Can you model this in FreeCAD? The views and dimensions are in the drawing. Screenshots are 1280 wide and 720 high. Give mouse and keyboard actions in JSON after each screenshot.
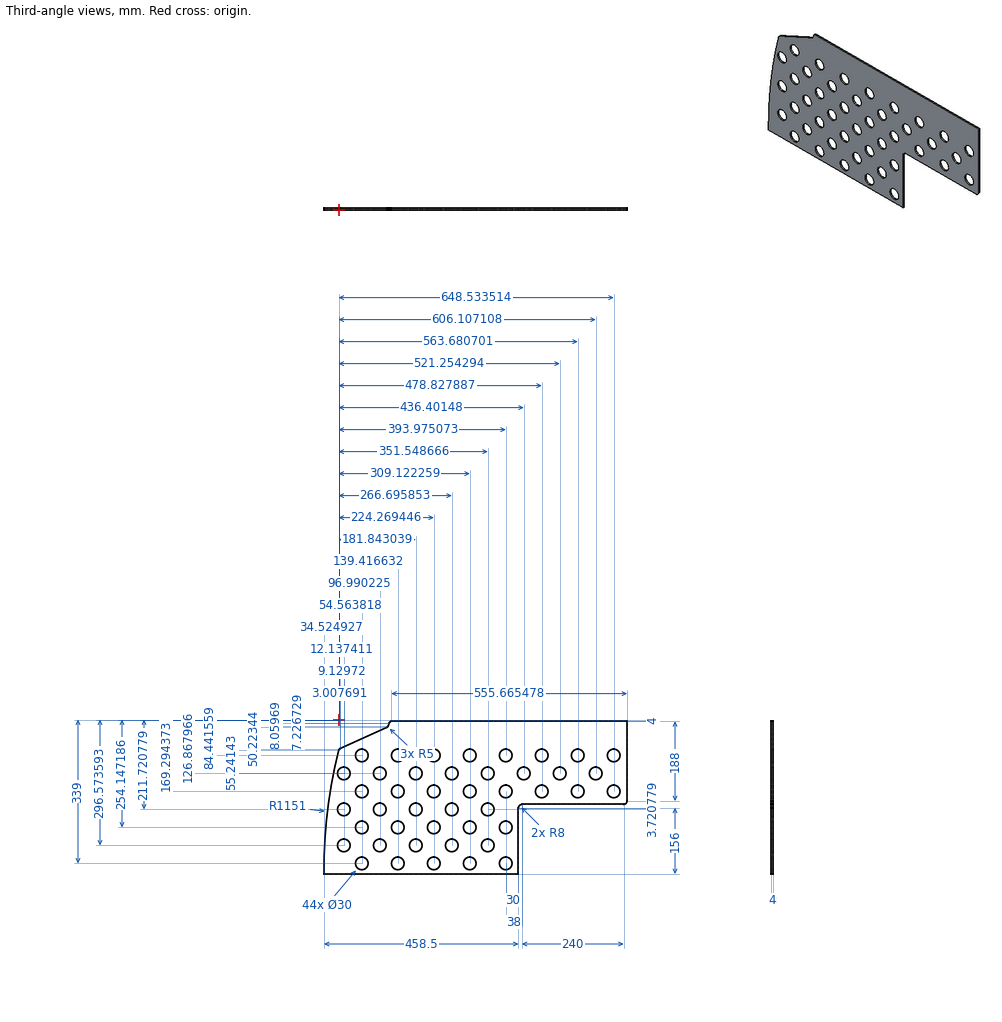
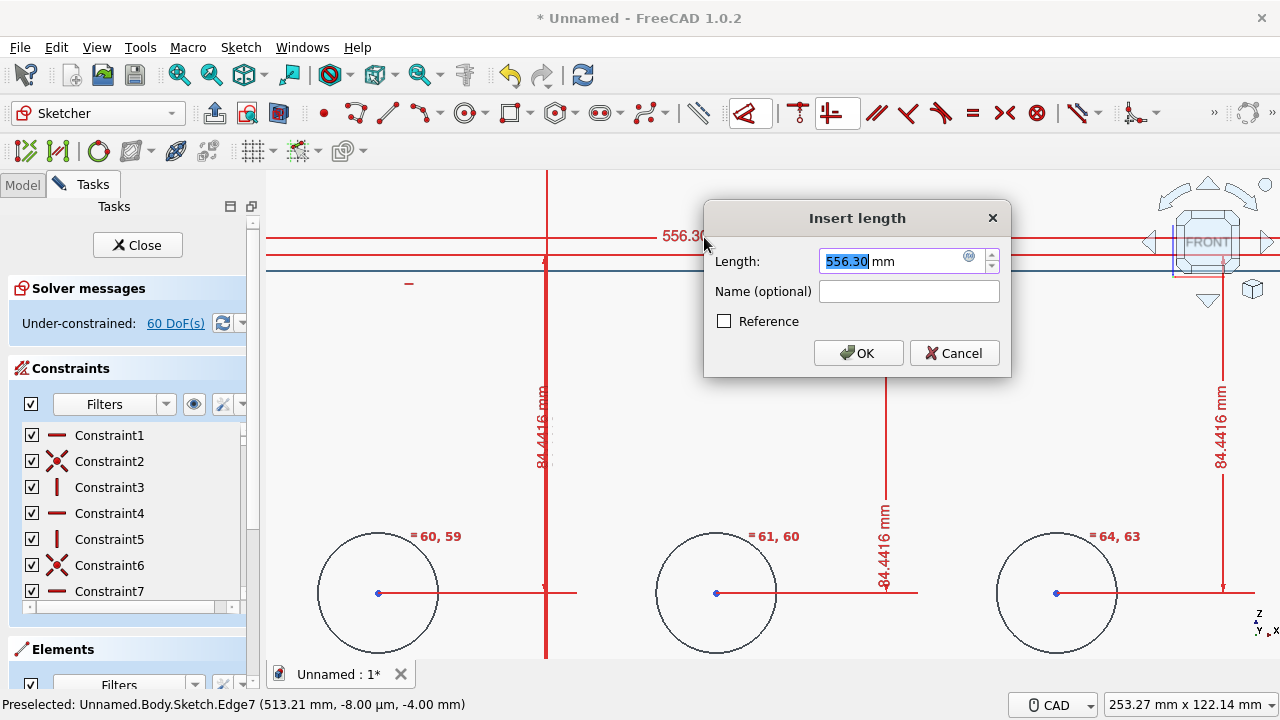
{"action": "type", "text": "555.665478"}
{"action": "key", "text": "Return"}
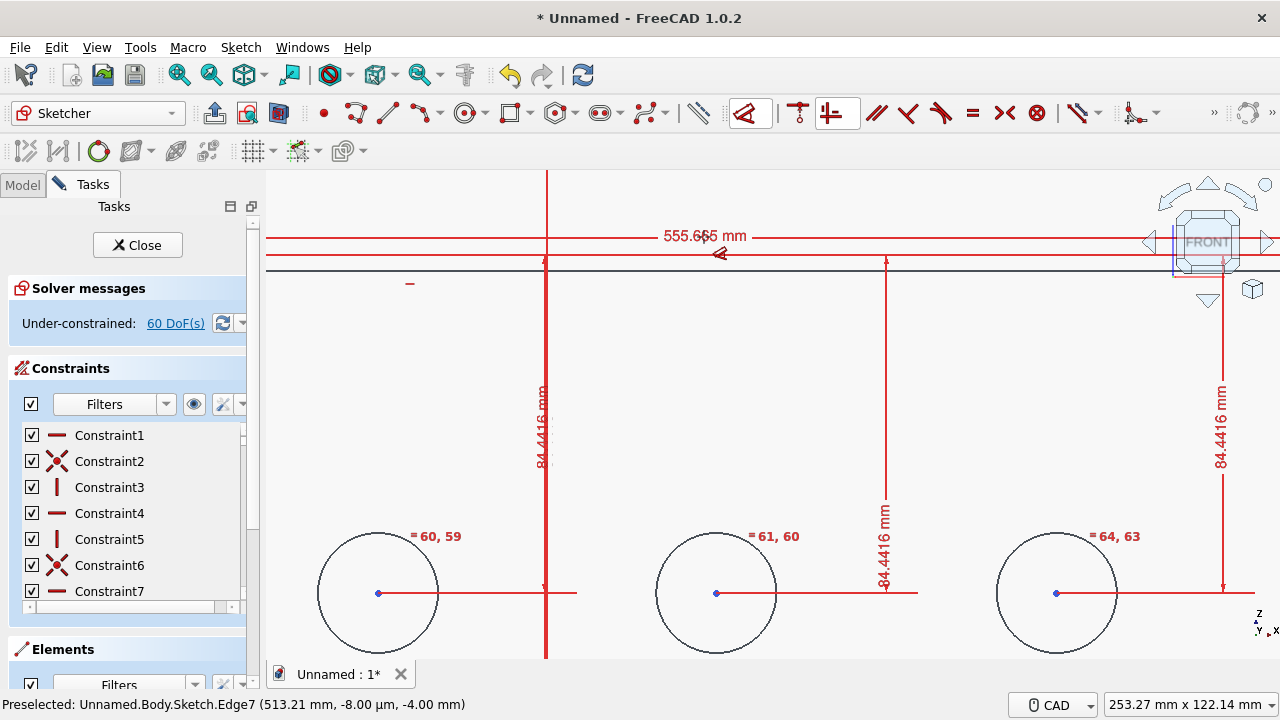
{"action": "scroll", "coordinate": [859, 271], "scroll_direction": "down", "scroll_amount": 8}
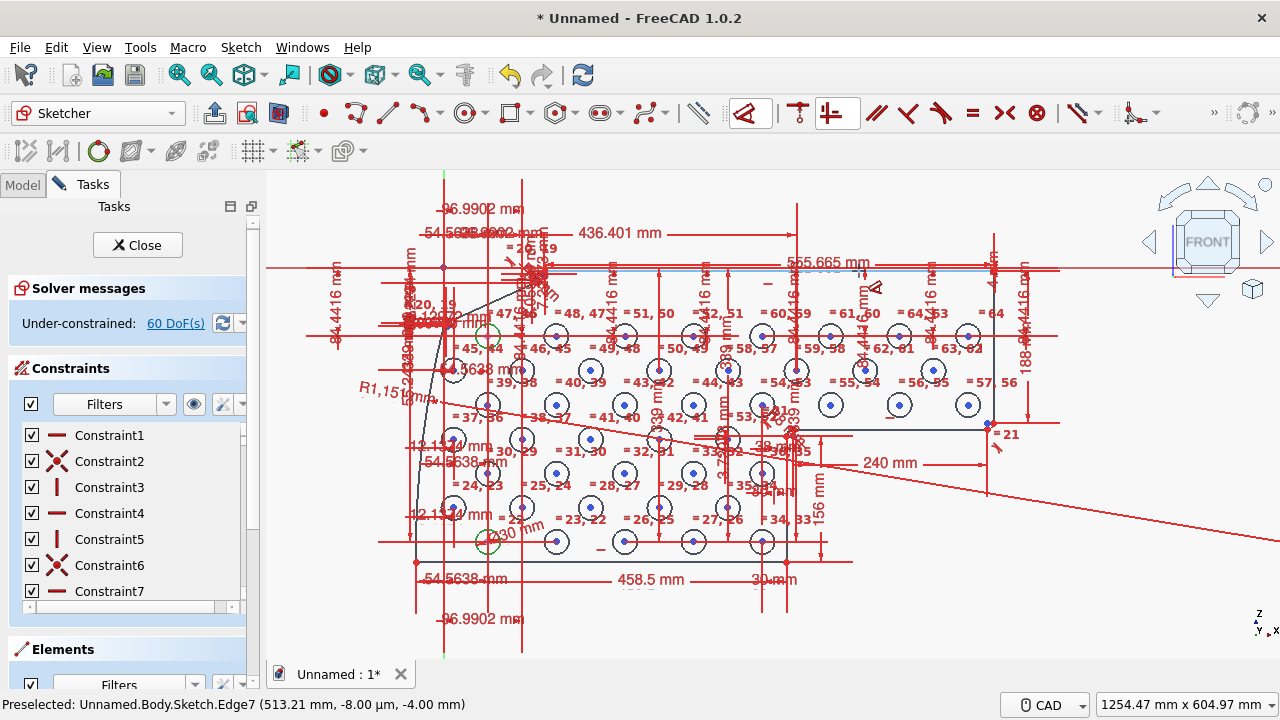
{"action": "scroll", "coordinate": [416, 562], "scroll_direction": "up", "scroll_amount": 2}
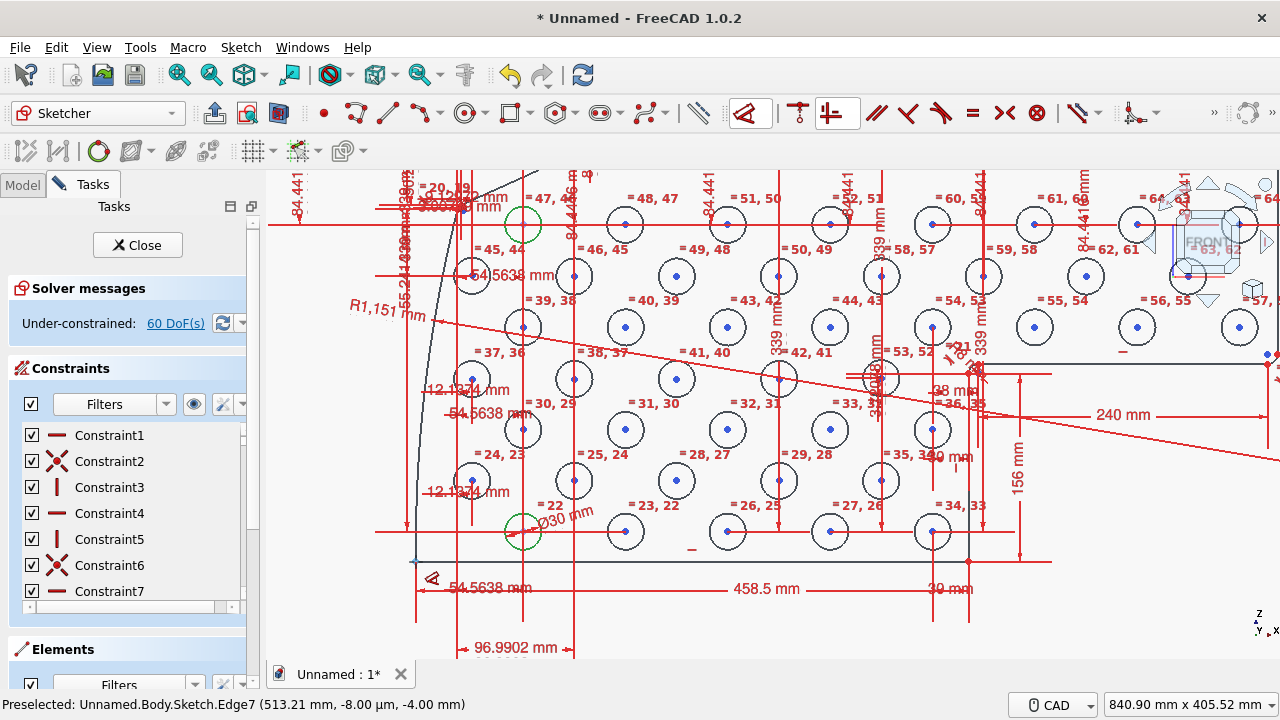
{"action": "left_click", "coordinate": [416, 562]}
{"action": "left_click", "coordinate": [437, 620]}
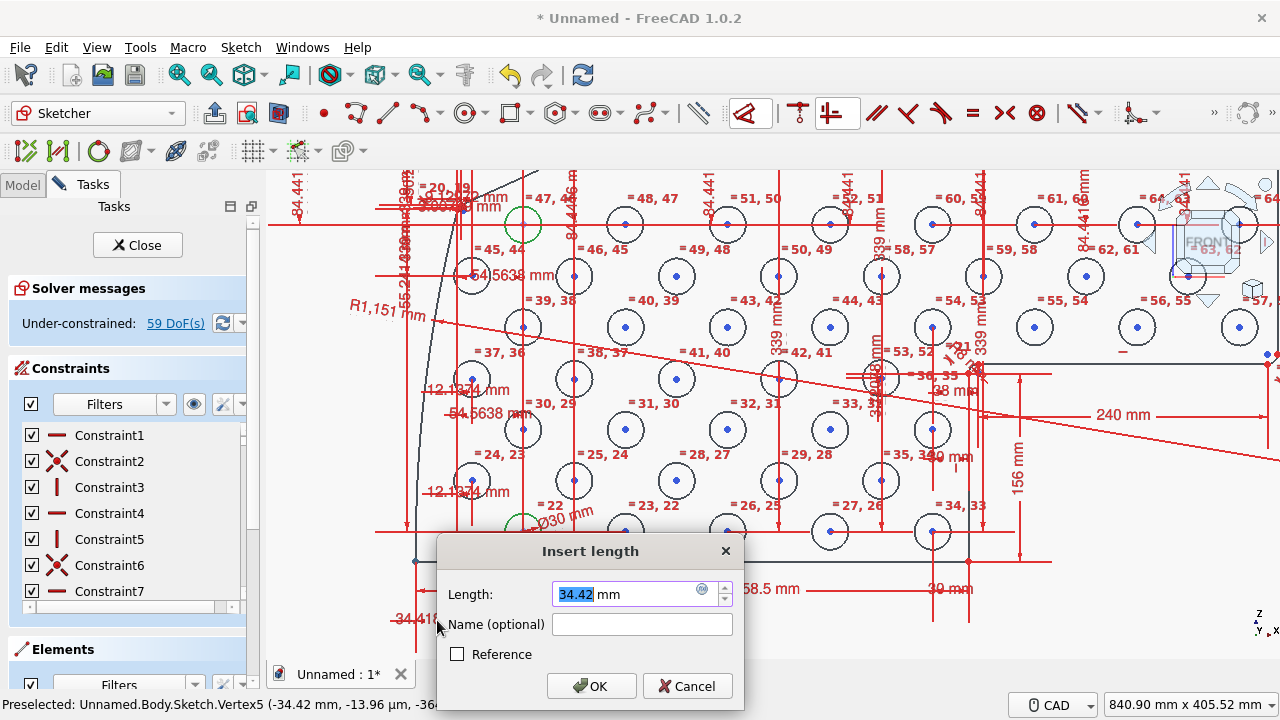
{"action": "type", "text": "34.524927"}
{"action": "key", "text": "Return"}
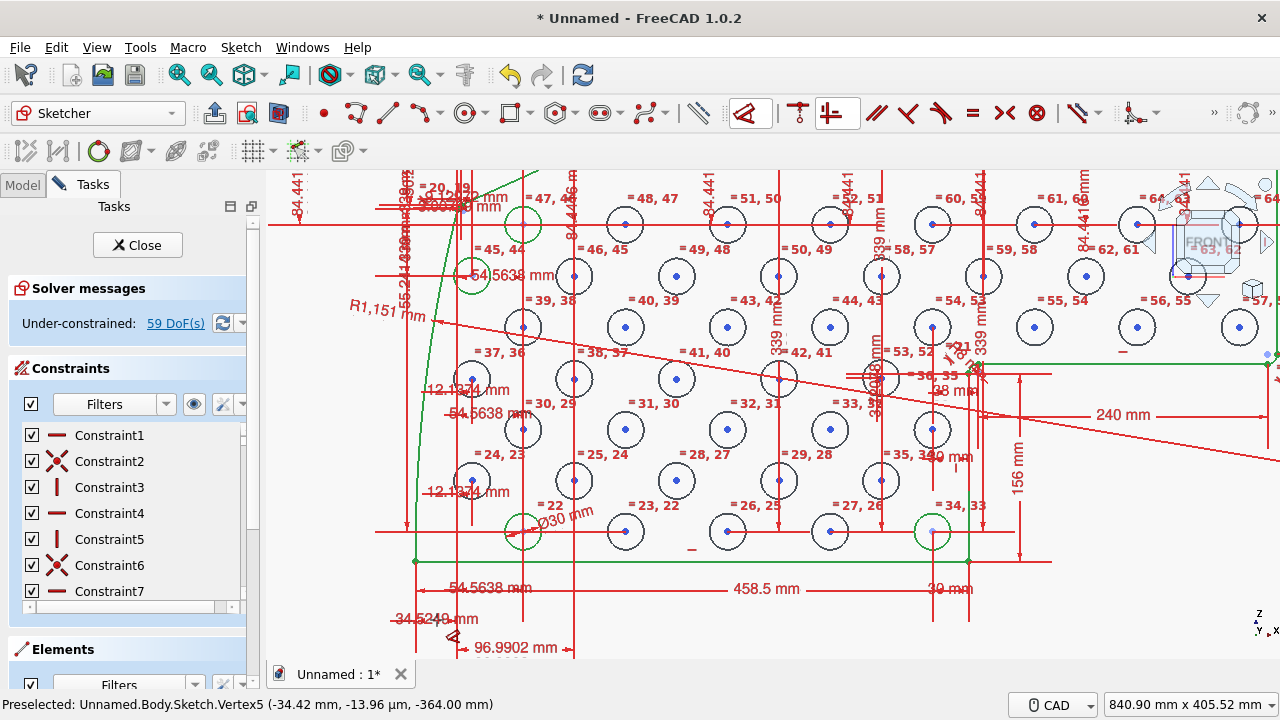
{"action": "left_click", "coordinate": [626, 532]}
{"action": "left_click", "coordinate": [580, 590]}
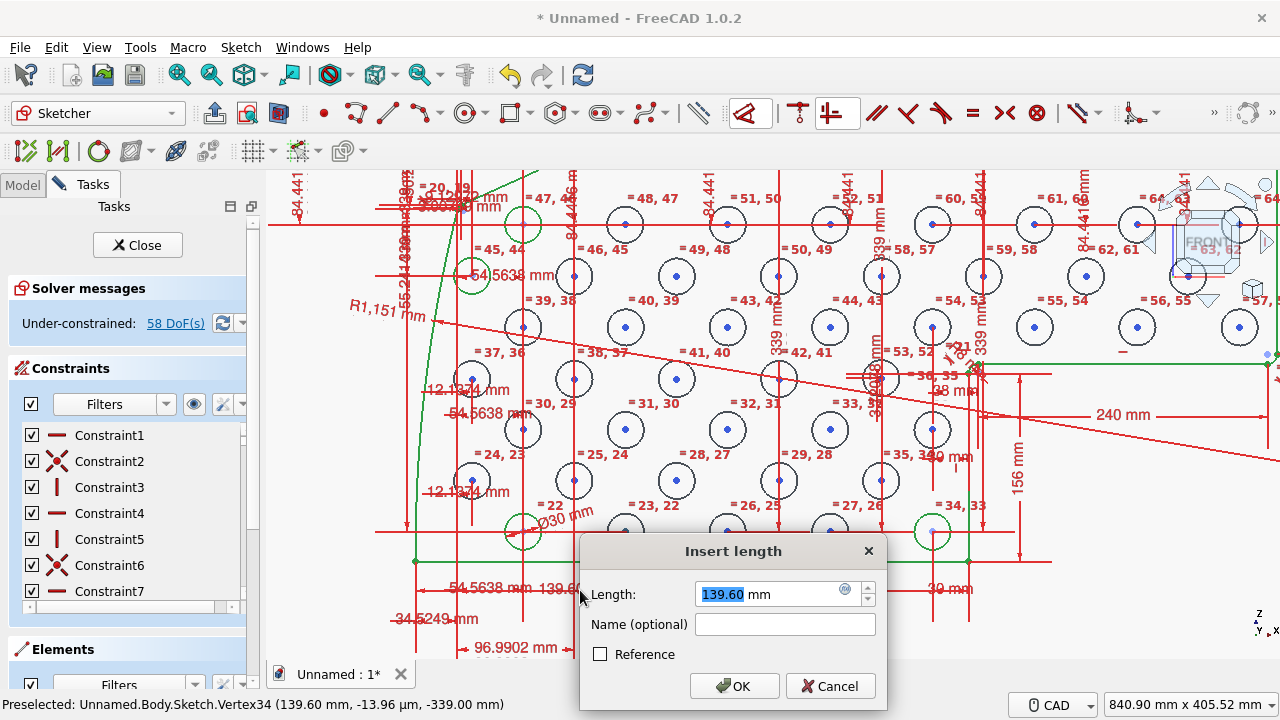
{"action": "type", "text": "139.416632"}
{"action": "key", "text": "Return"}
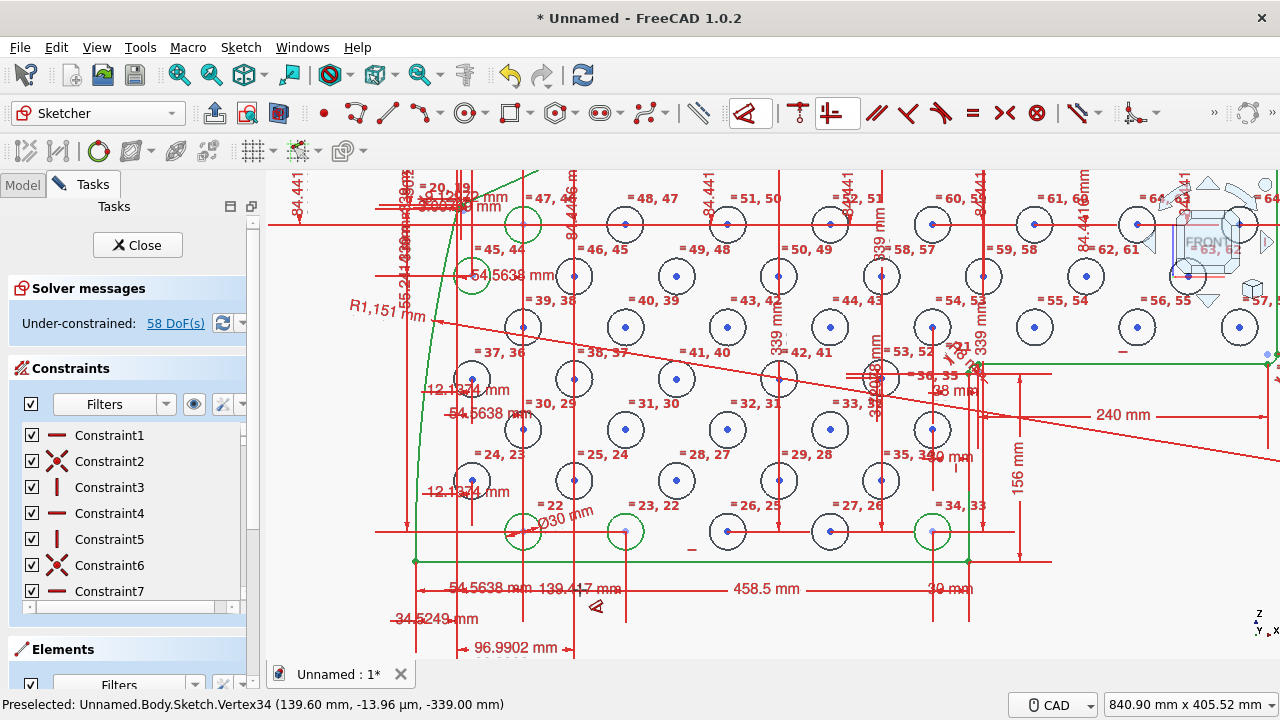
{"action": "left_click", "coordinate": [472, 481]}
{"action": "left_click", "coordinate": [399, 339]}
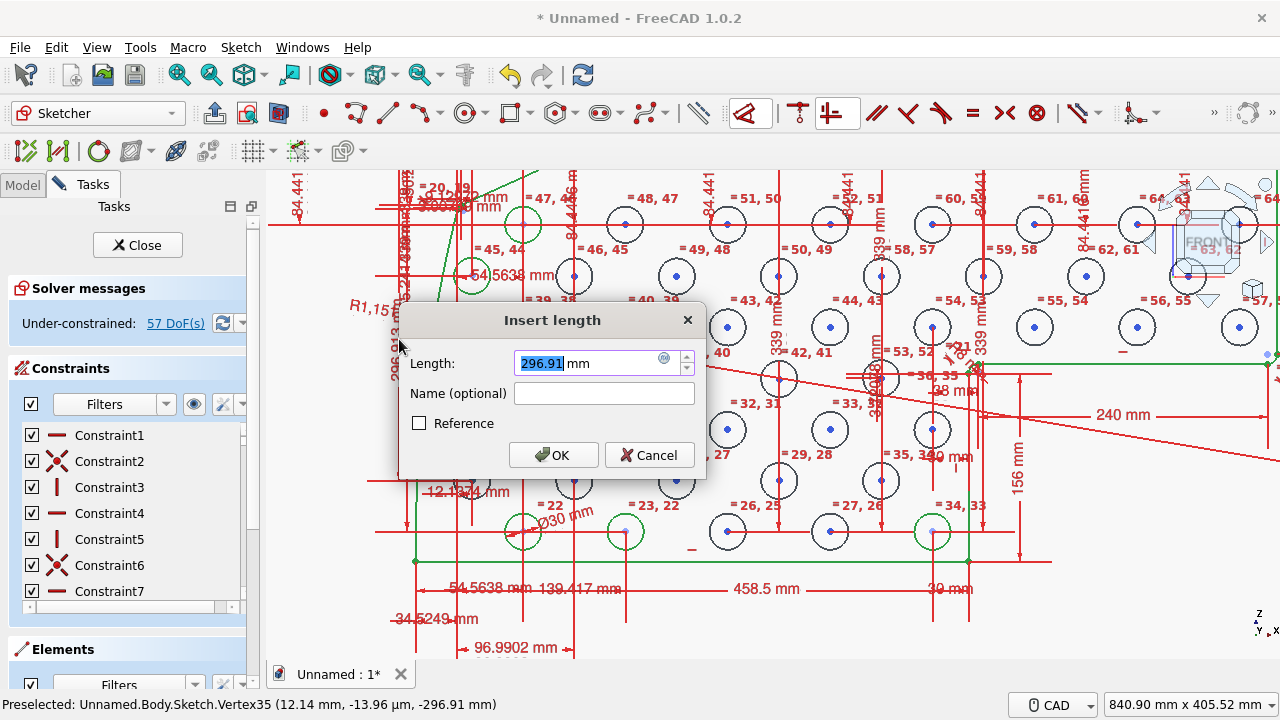
{"action": "type", "text": "296.573593"}
{"action": "key", "text": "Return"}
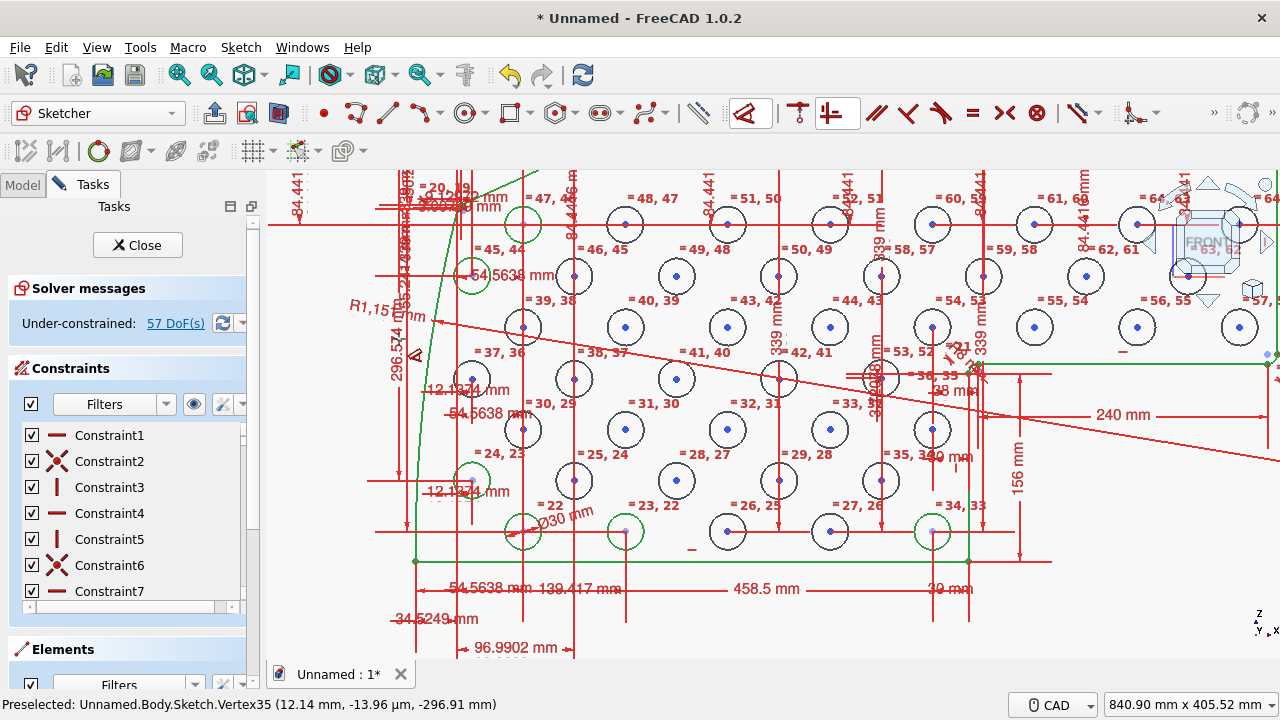
{"action": "left_click", "coordinate": [574, 481]}
{"action": "left_click", "coordinate": [608, 274]}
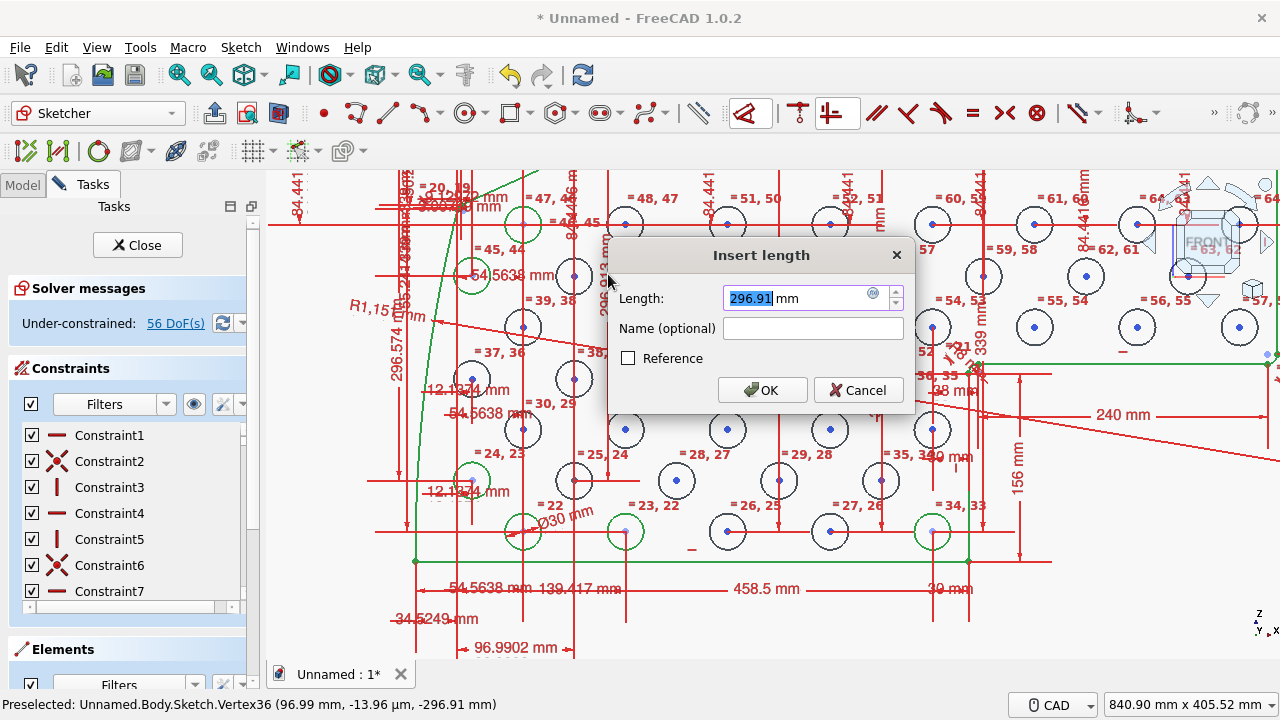
{"action": "type", "text": "296.573593"}
{"action": "key", "text": "Return"}